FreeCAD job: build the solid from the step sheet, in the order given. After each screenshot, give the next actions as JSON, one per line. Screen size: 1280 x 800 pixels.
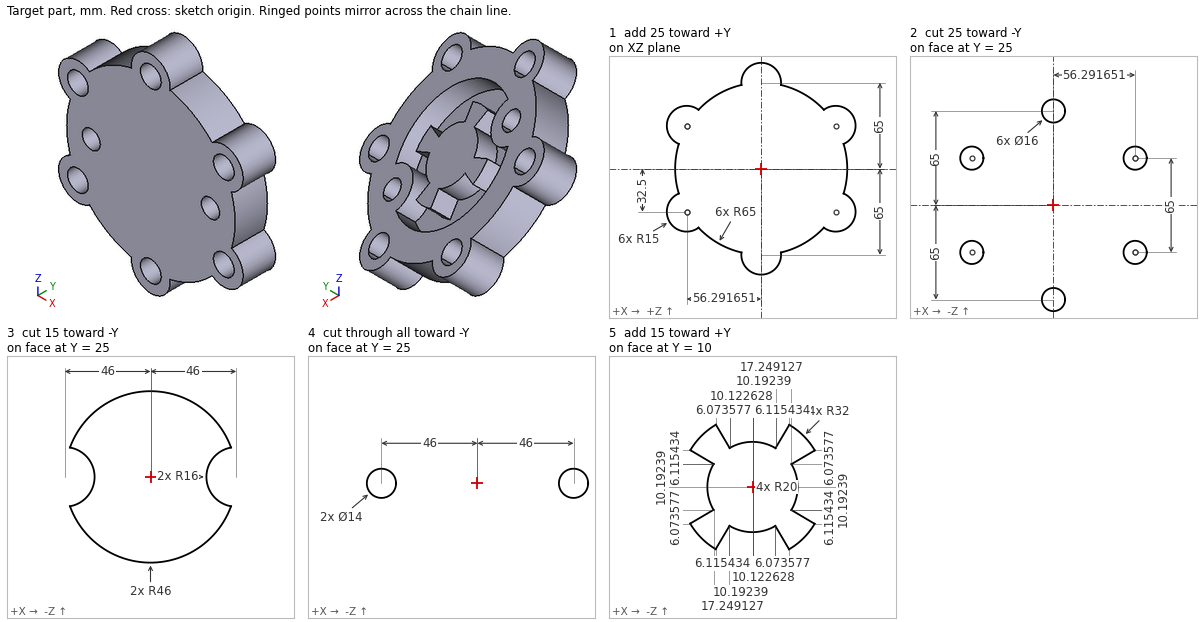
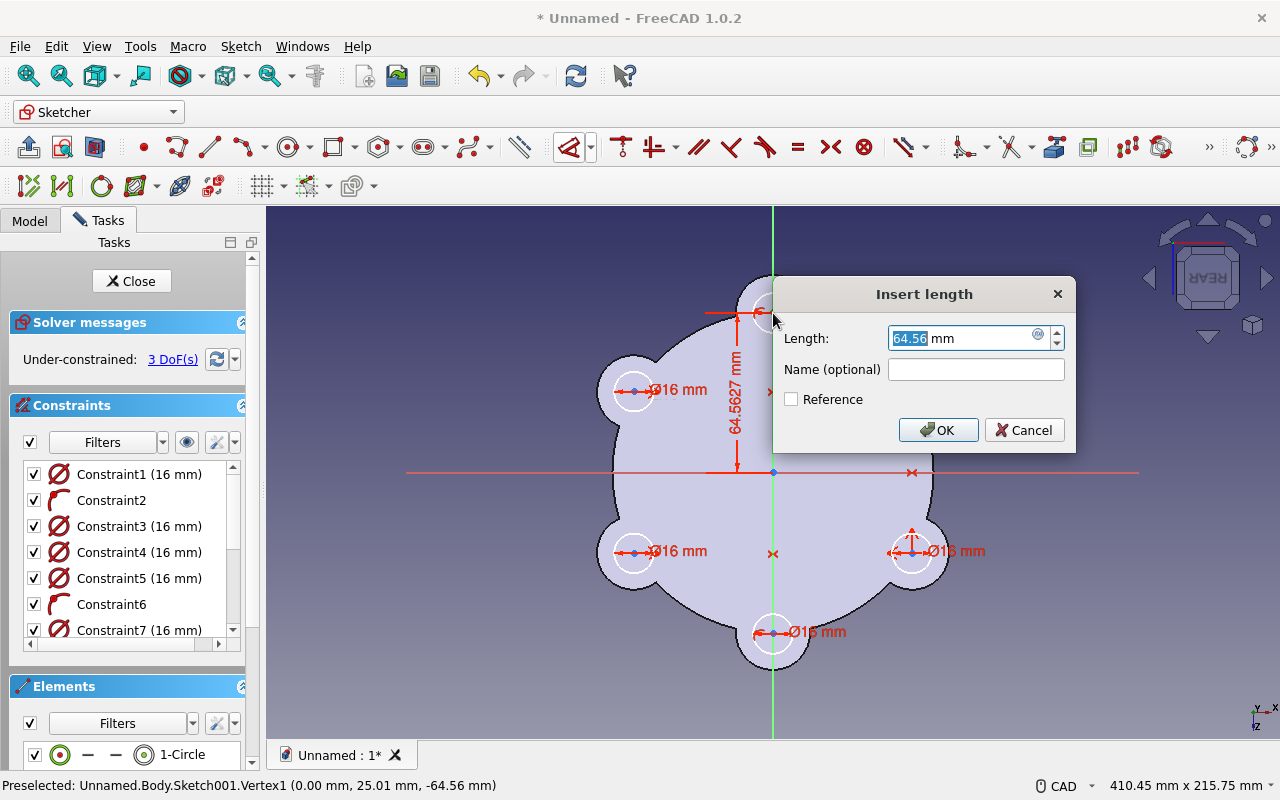
{"action": "type", "text": "65"}
{"action": "key", "text": "Return"}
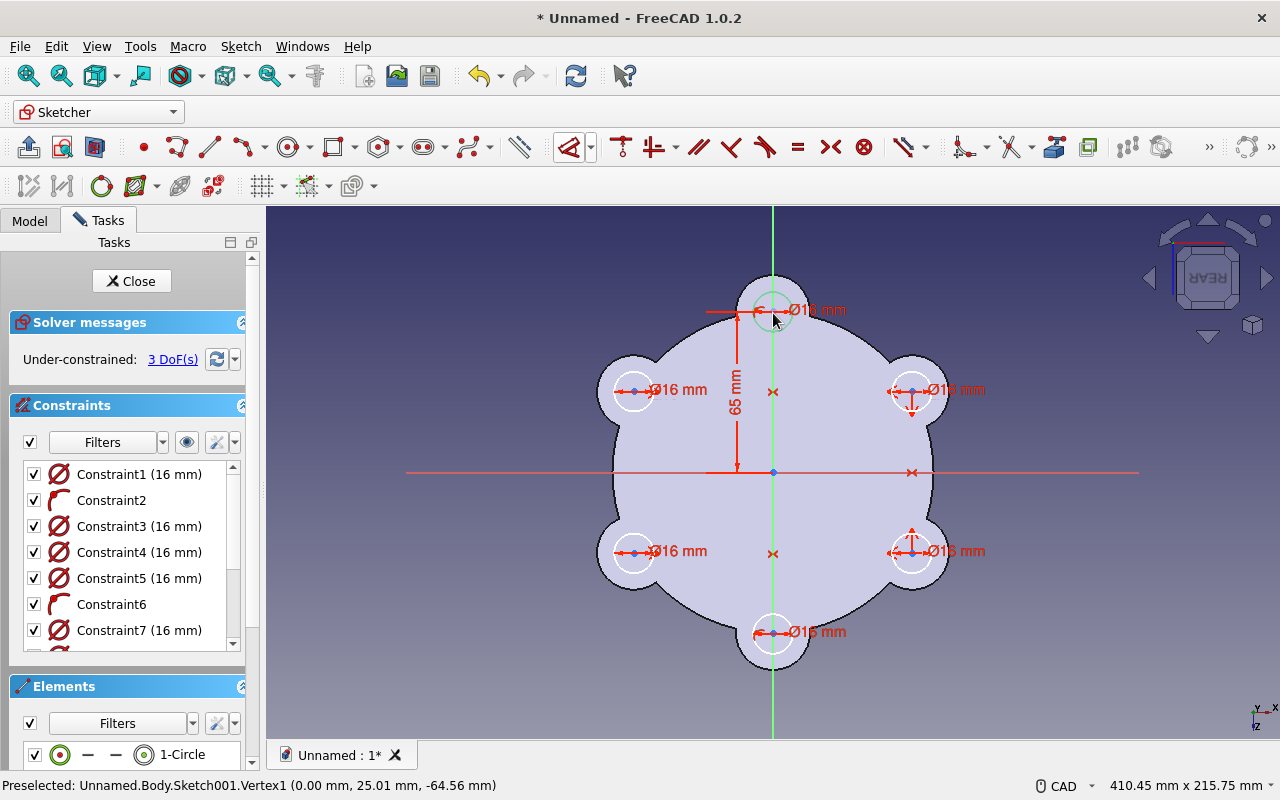
{"action": "left_click", "coordinate": [773, 634]}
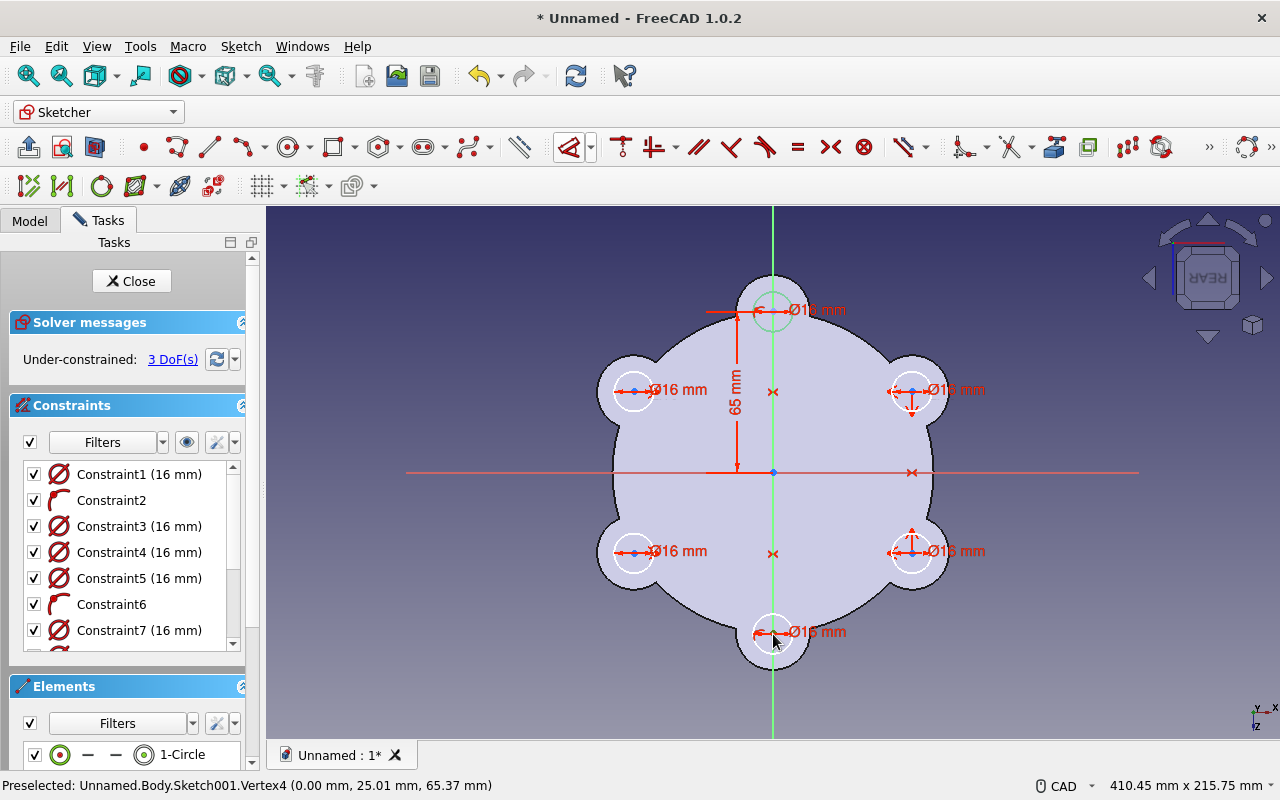
{"action": "key", "text": "i"}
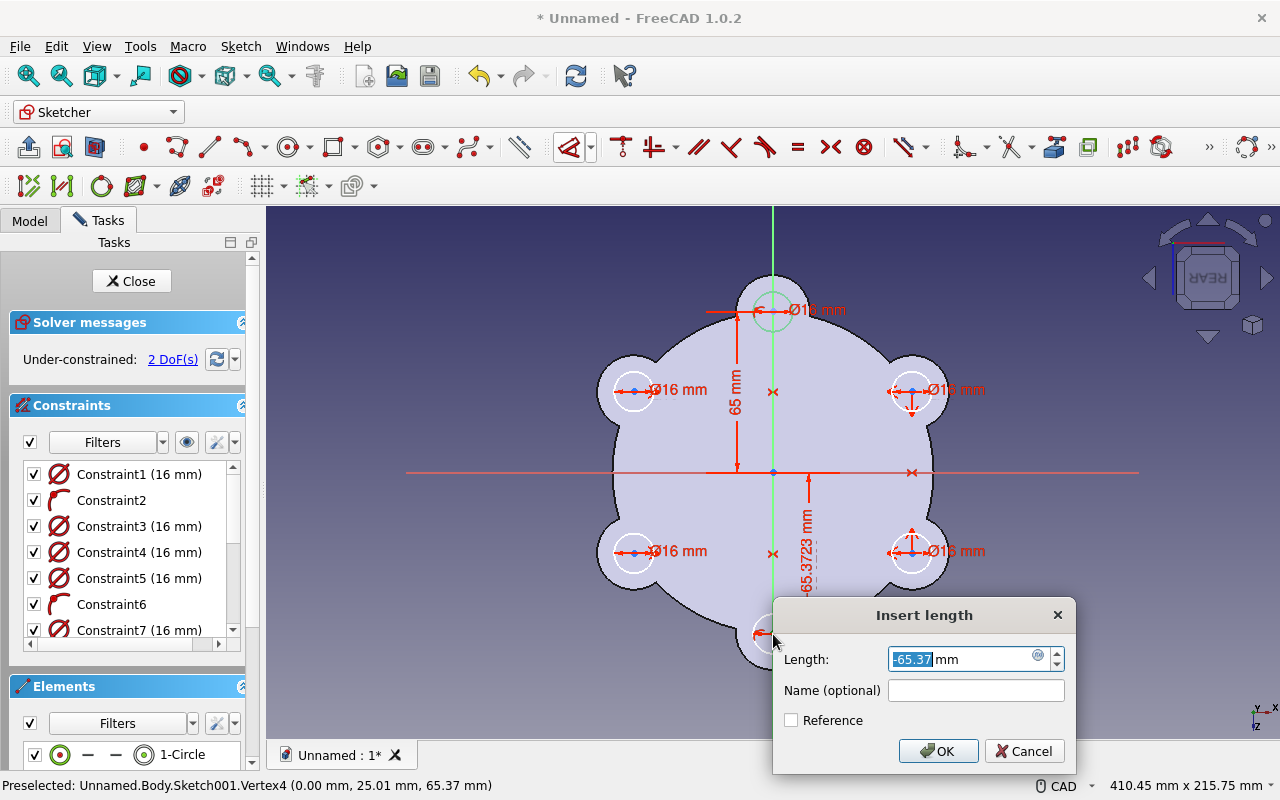
{"action": "type", "text": "-65"}
{"action": "key", "text": "Return"}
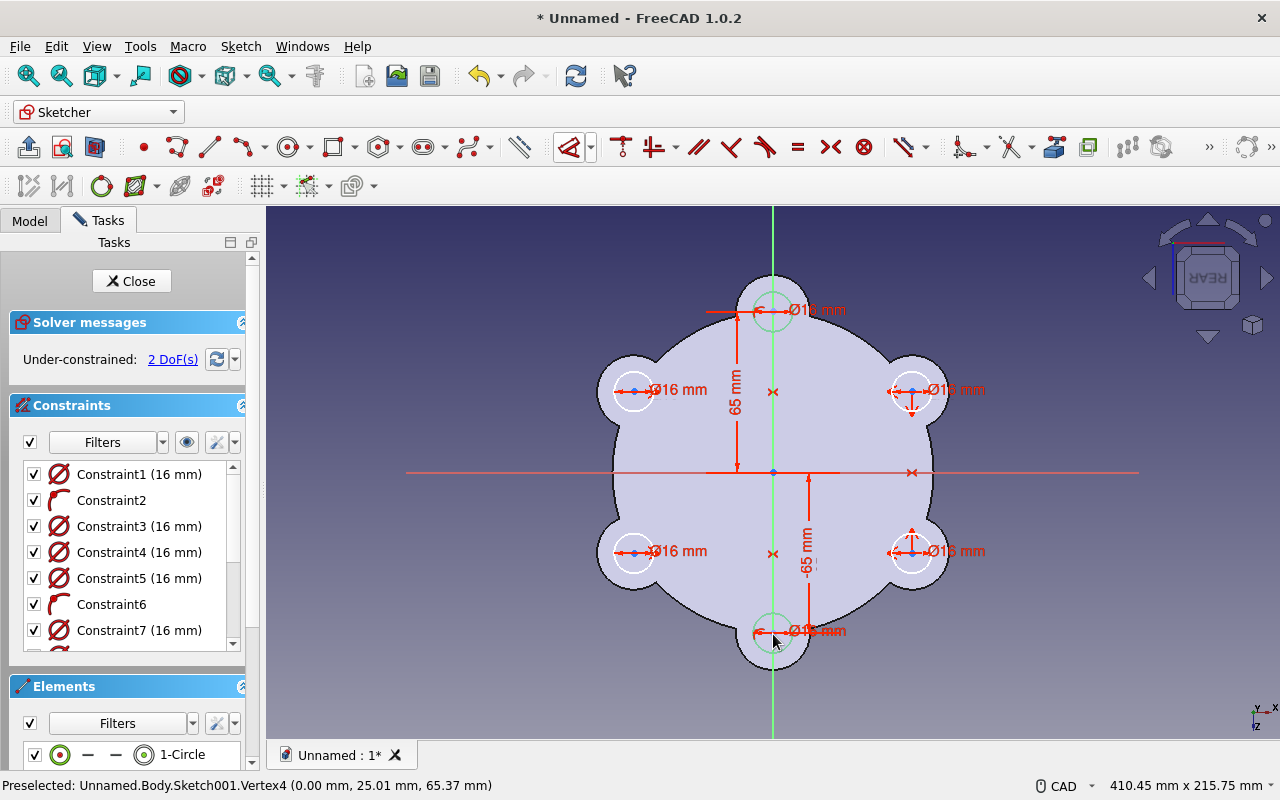
{"action": "left_click", "coordinate": [912, 392]}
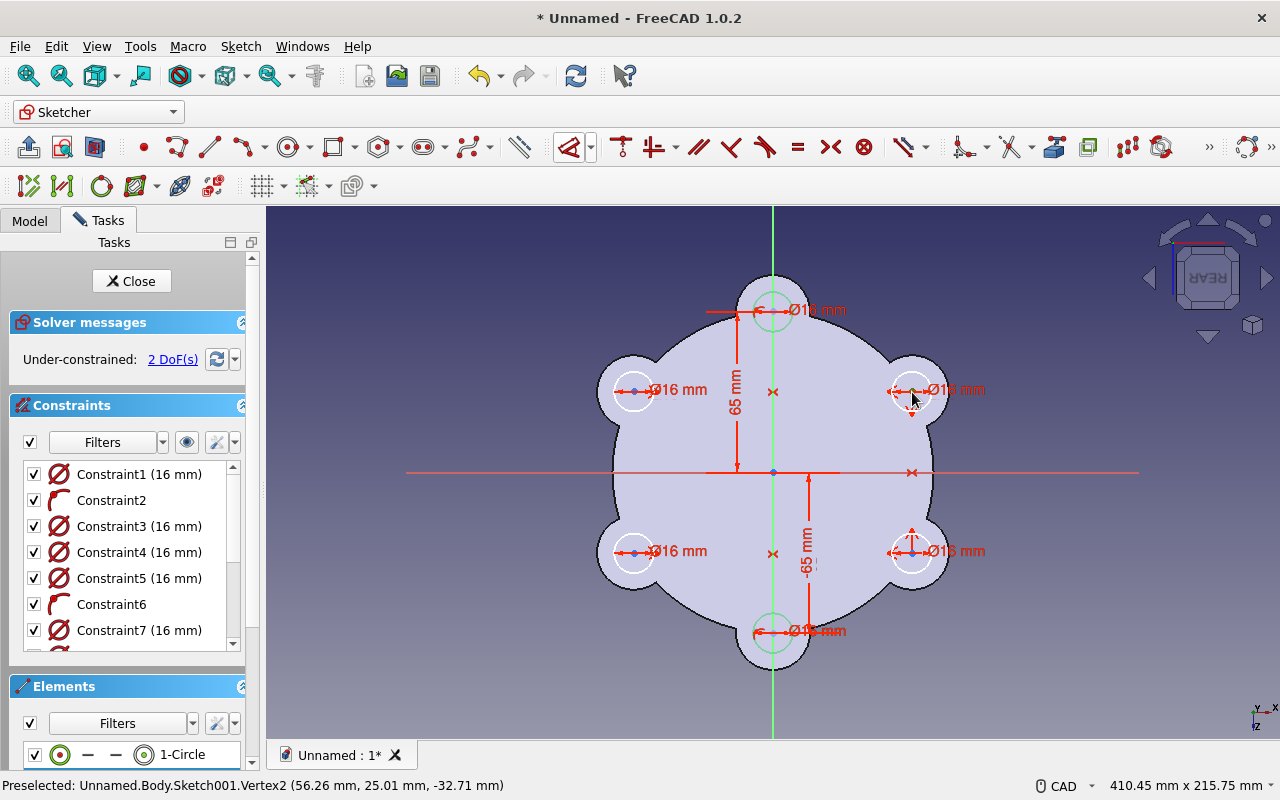
{"action": "left_click", "coordinate": [912, 553]}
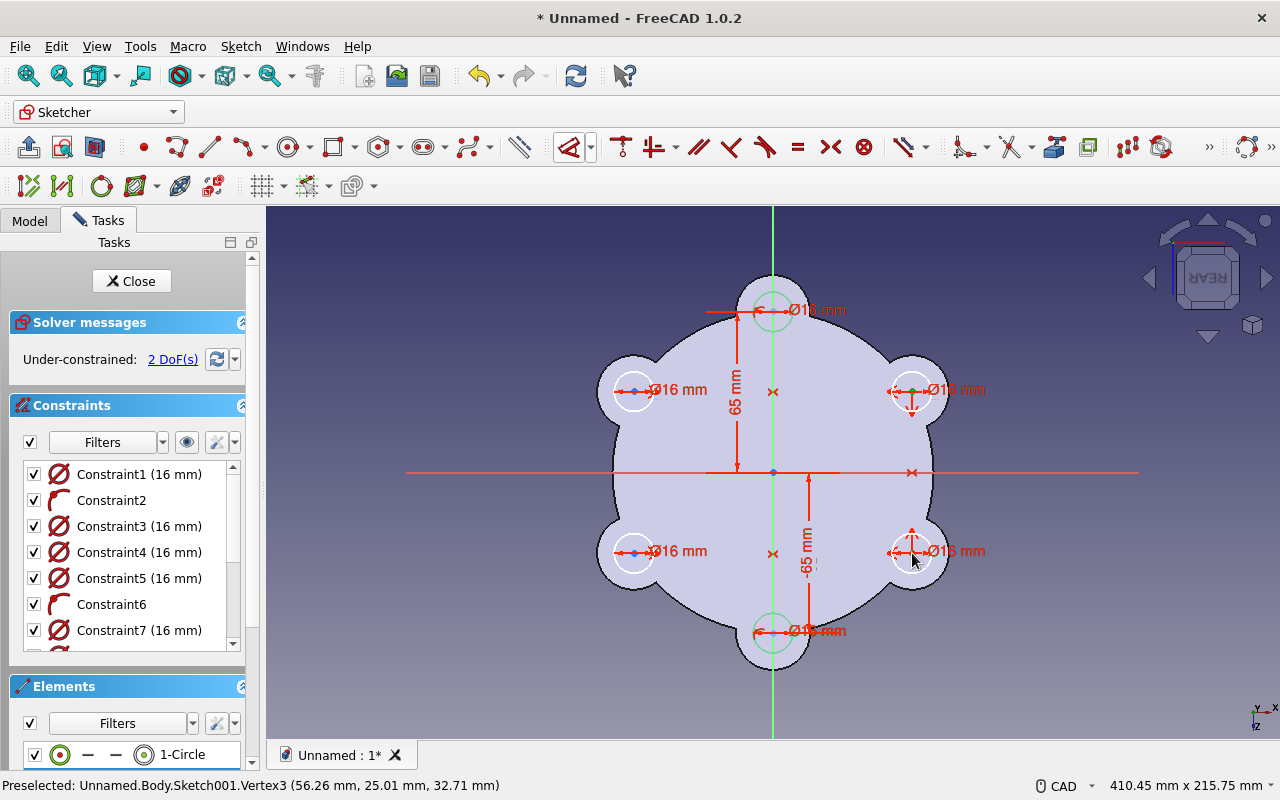
{"action": "key", "text": "i"}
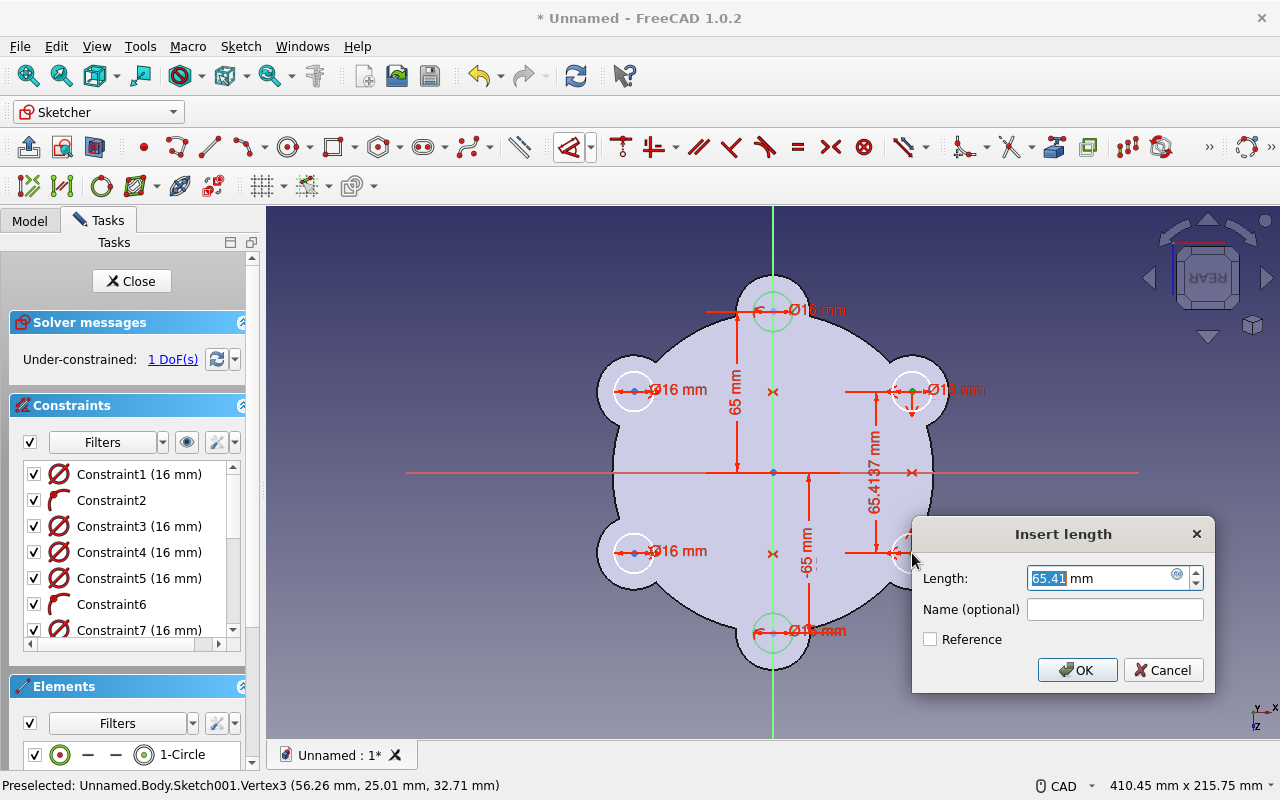
{"action": "type", "text": "65"}
{"action": "key", "text": "Return"}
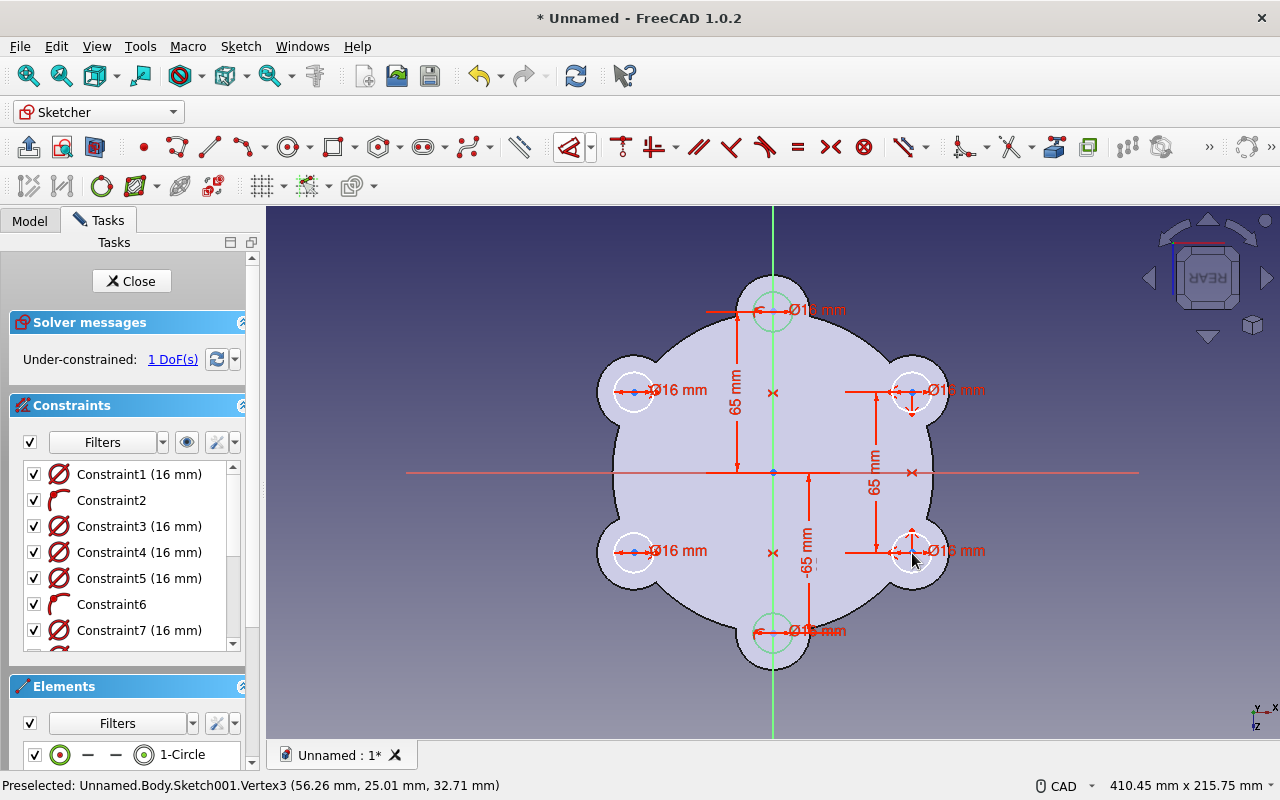
{"action": "left_click", "coordinate": [912, 392]}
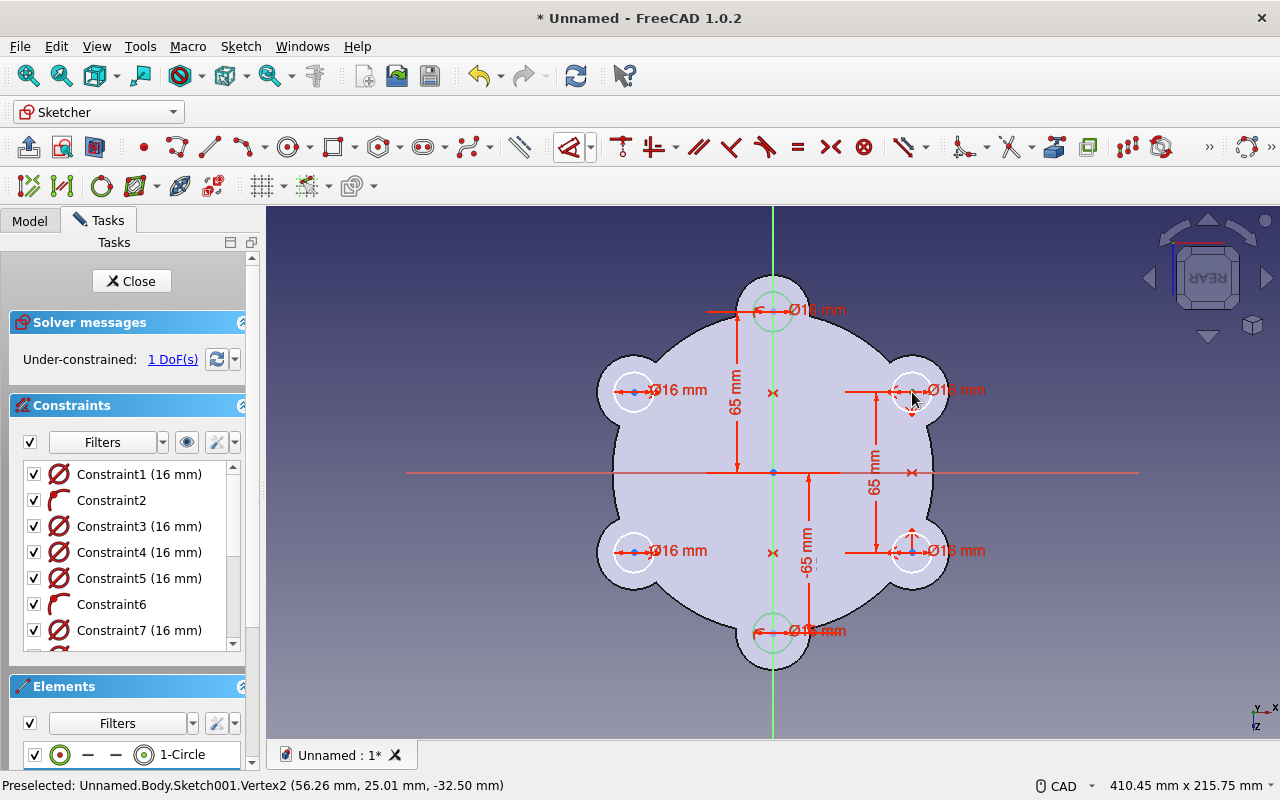
{"action": "left_click", "coordinate": [590, 148]}